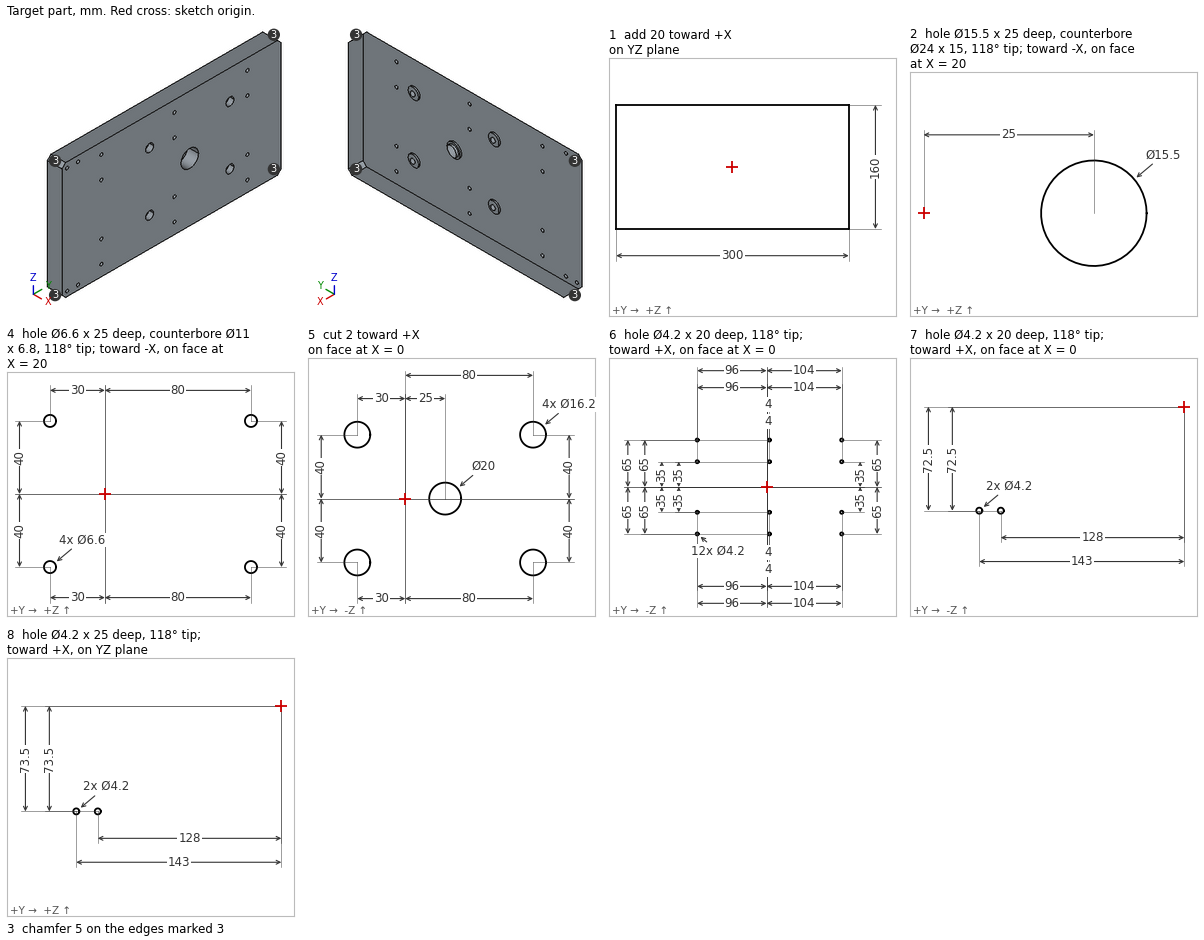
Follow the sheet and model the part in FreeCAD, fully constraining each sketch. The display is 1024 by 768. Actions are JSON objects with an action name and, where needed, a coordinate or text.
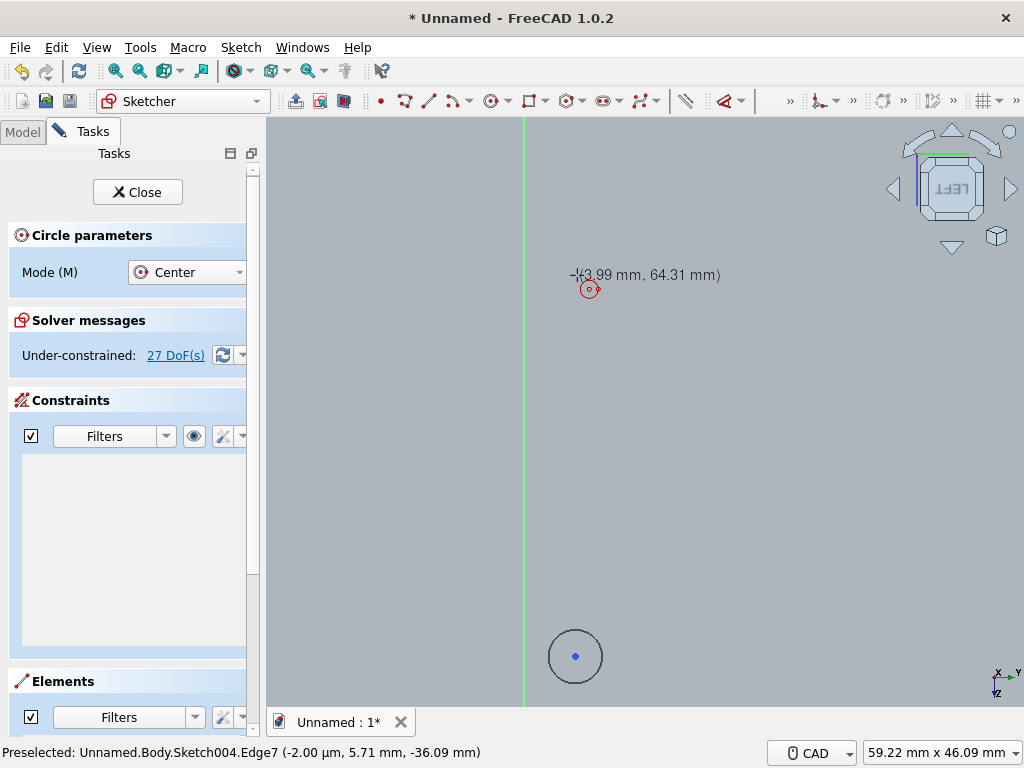
{"action": "scroll", "coordinate": [577, 275], "scroll_direction": "down", "scroll_amount": 9}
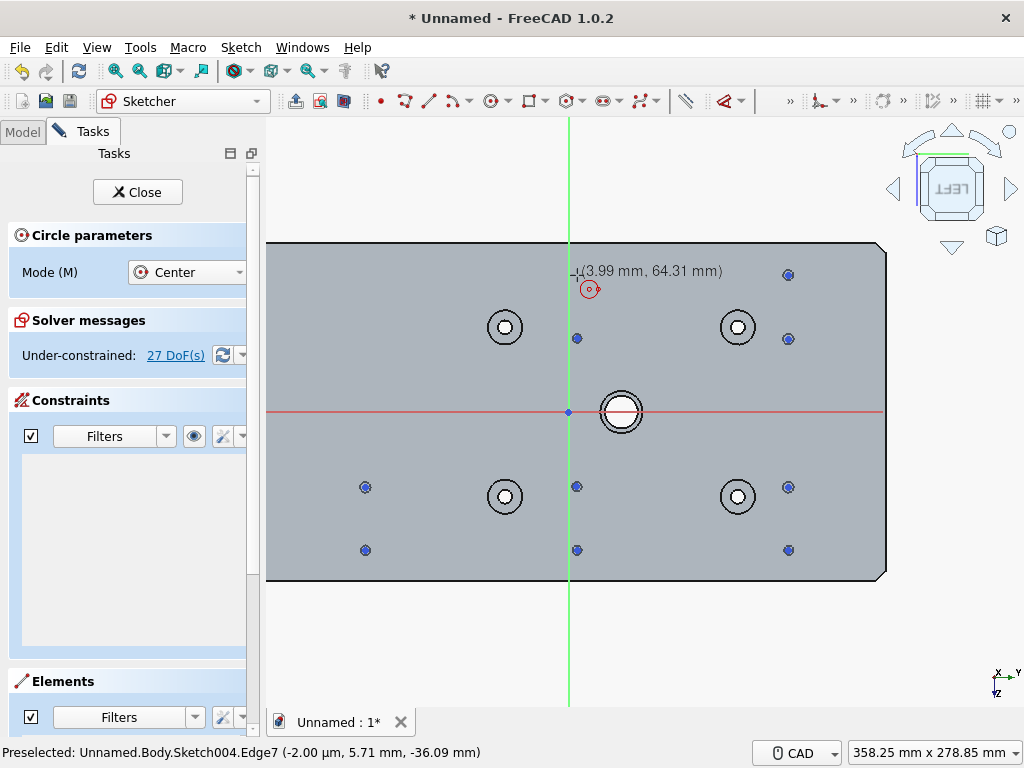
{"action": "scroll", "coordinate": [577, 275], "scroll_direction": "up", "scroll_amount": 4}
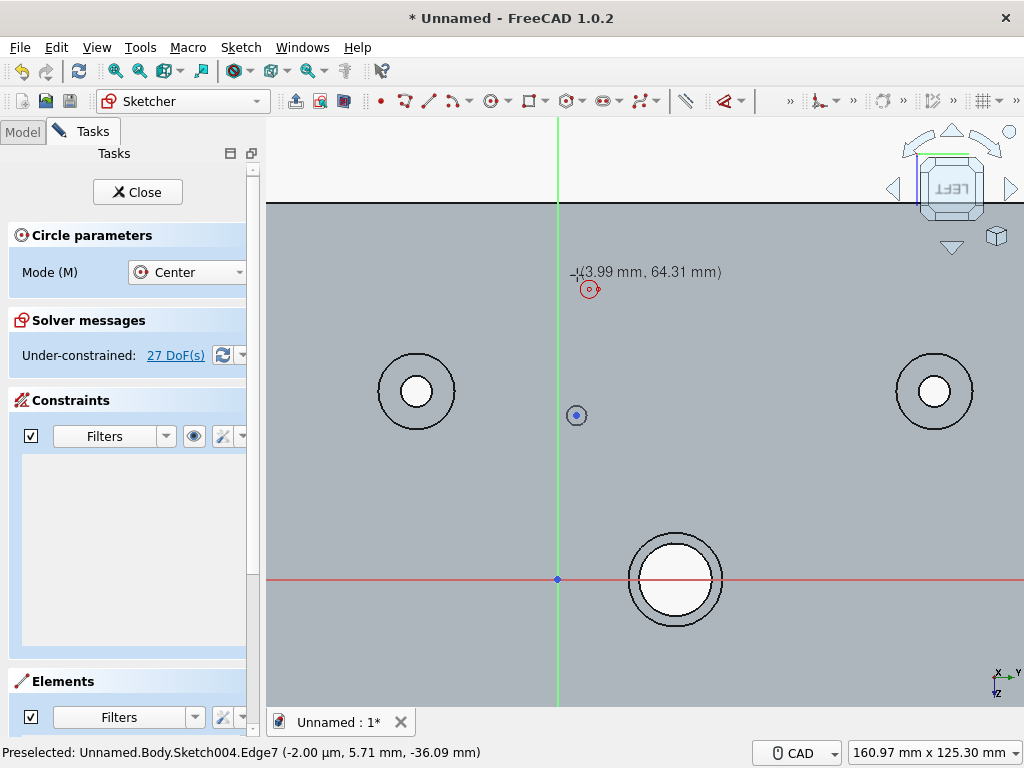
{"action": "left_click", "coordinate": [577, 274]}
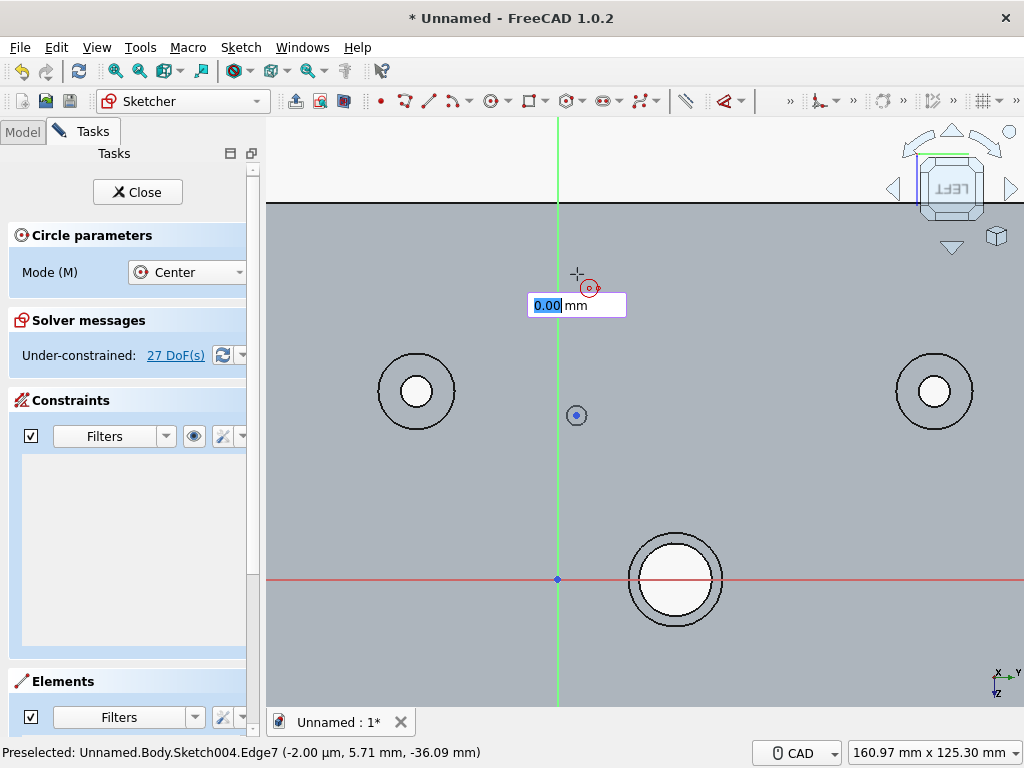
{"action": "scroll", "coordinate": [584, 267], "scroll_direction": "up", "scroll_amount": 3}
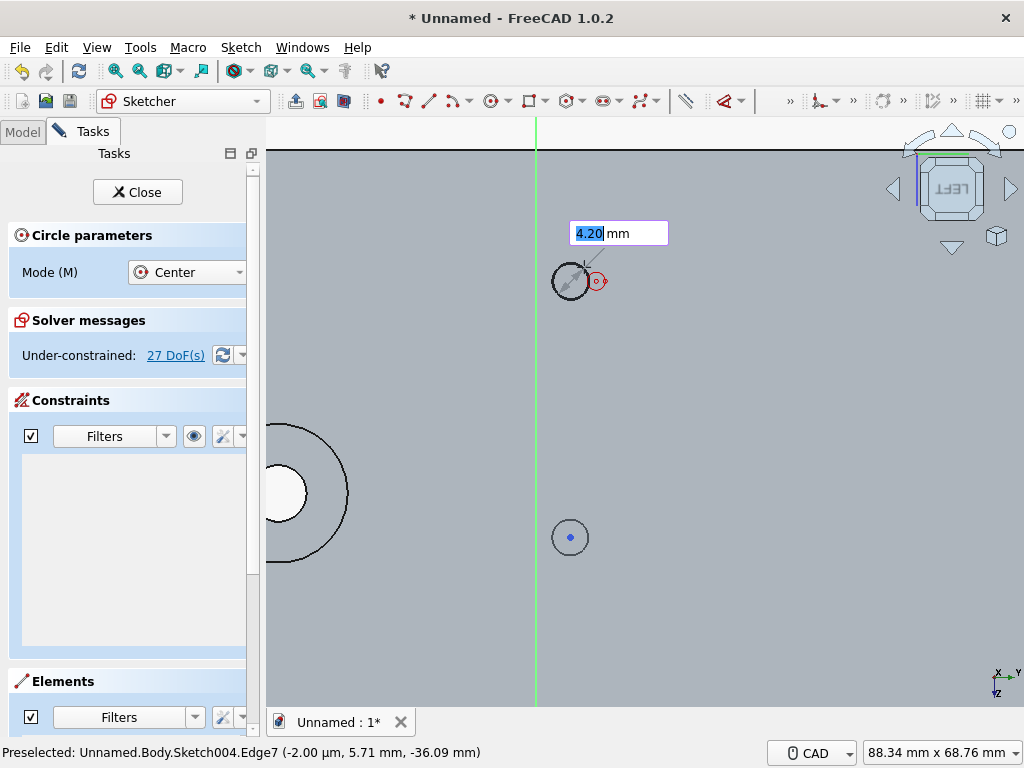
{"action": "left_click", "coordinate": [583, 266]}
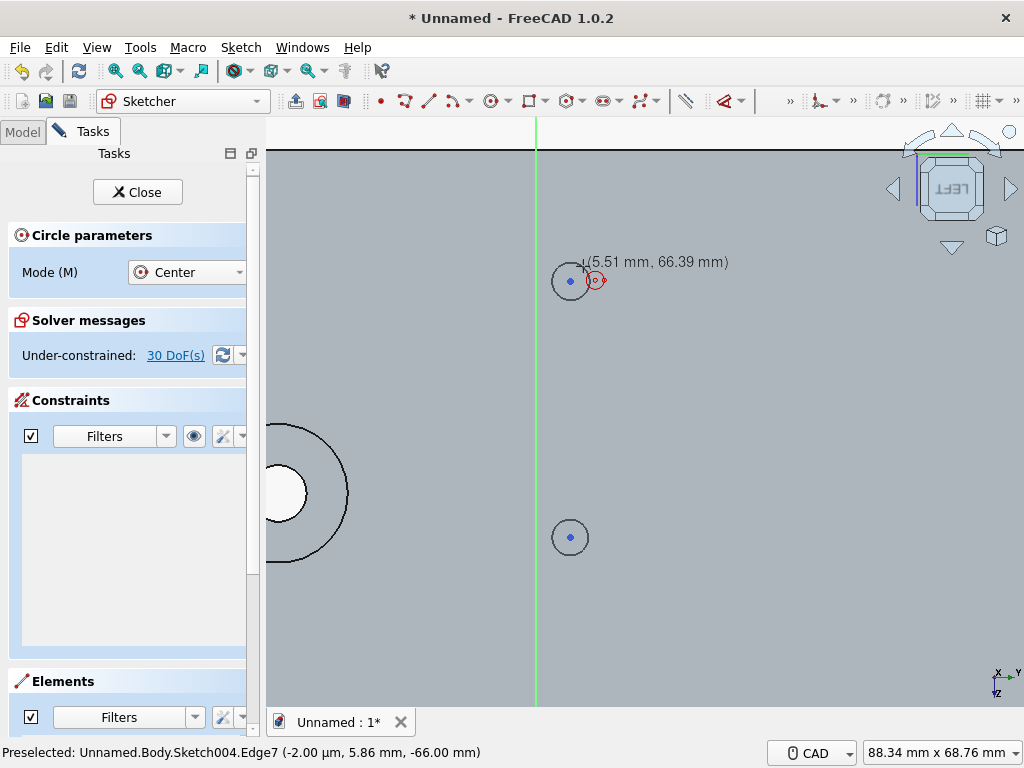
{"action": "scroll", "coordinate": [579, 273], "scroll_direction": "down", "scroll_amount": 7}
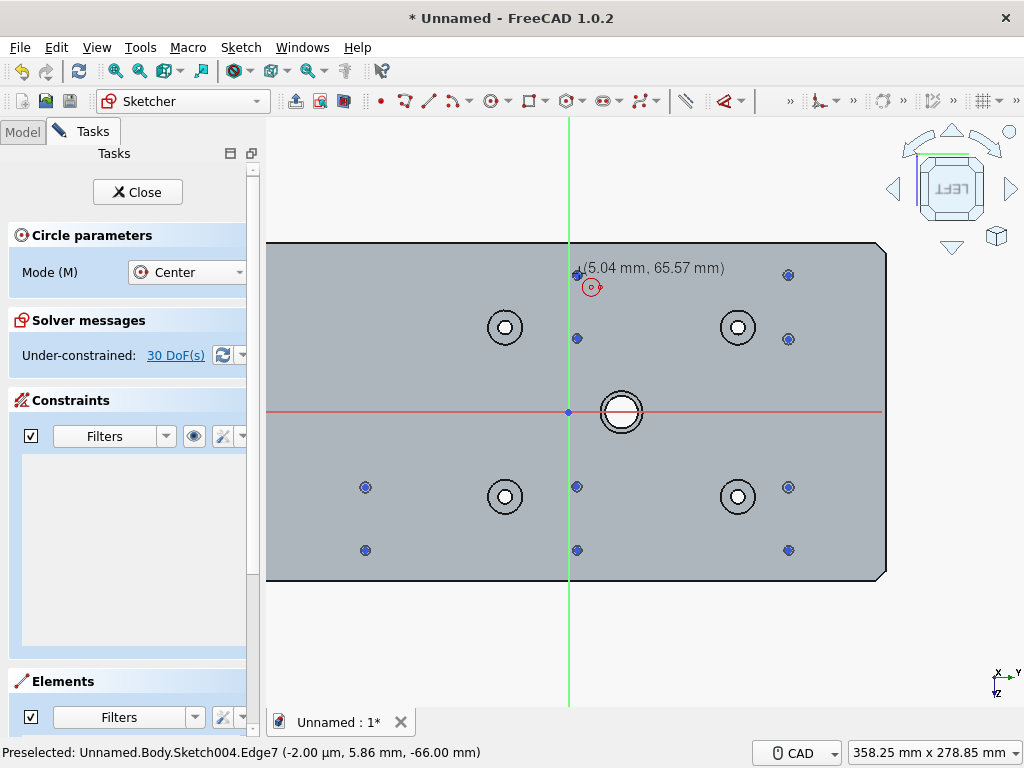
{"action": "scroll", "coordinate": [366, 338], "scroll_direction": "up", "scroll_amount": 9}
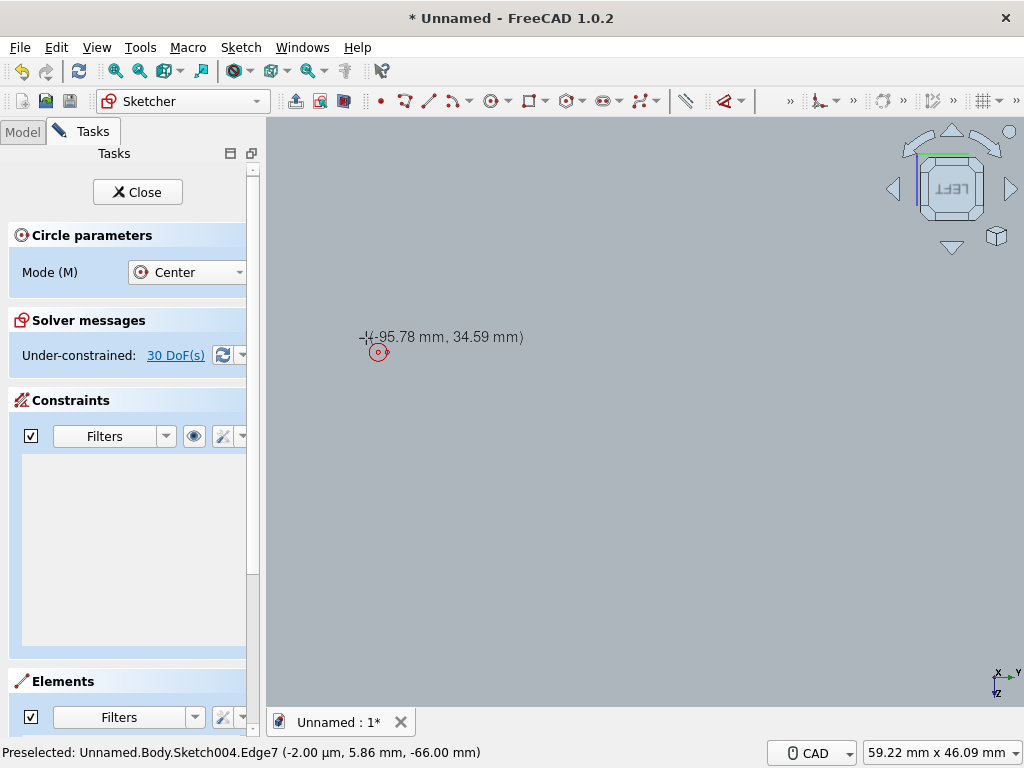
{"action": "scroll", "coordinate": [365, 338], "scroll_direction": "down", "scroll_amount": 9}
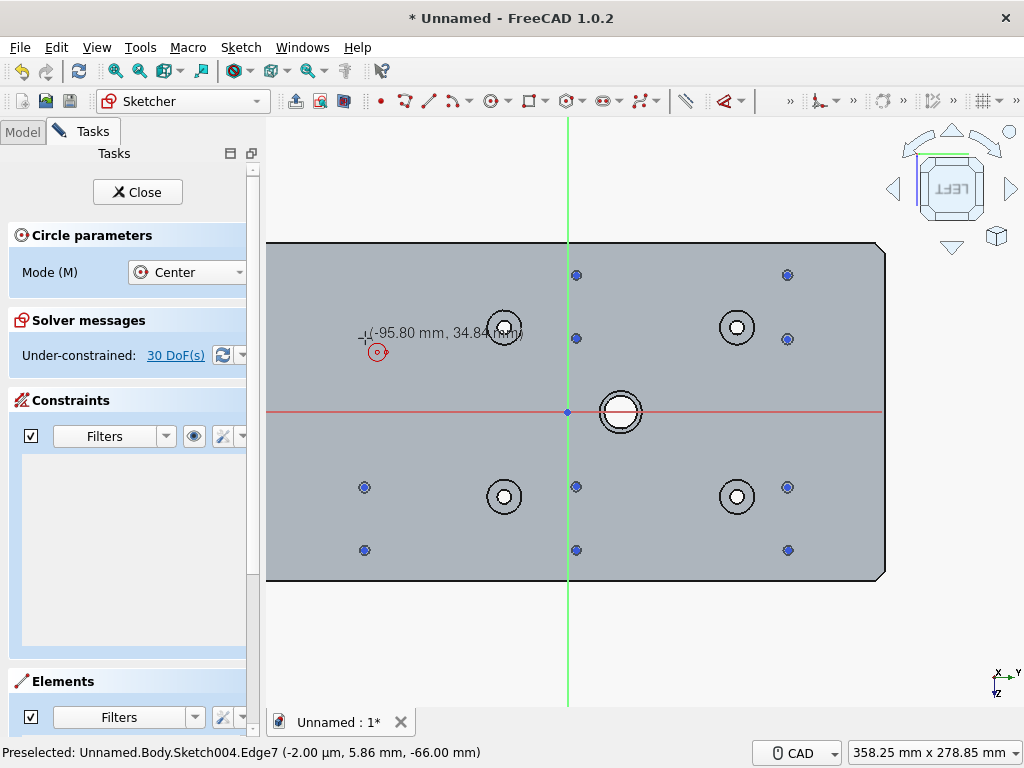
{"action": "left_click", "coordinate": [365, 338]}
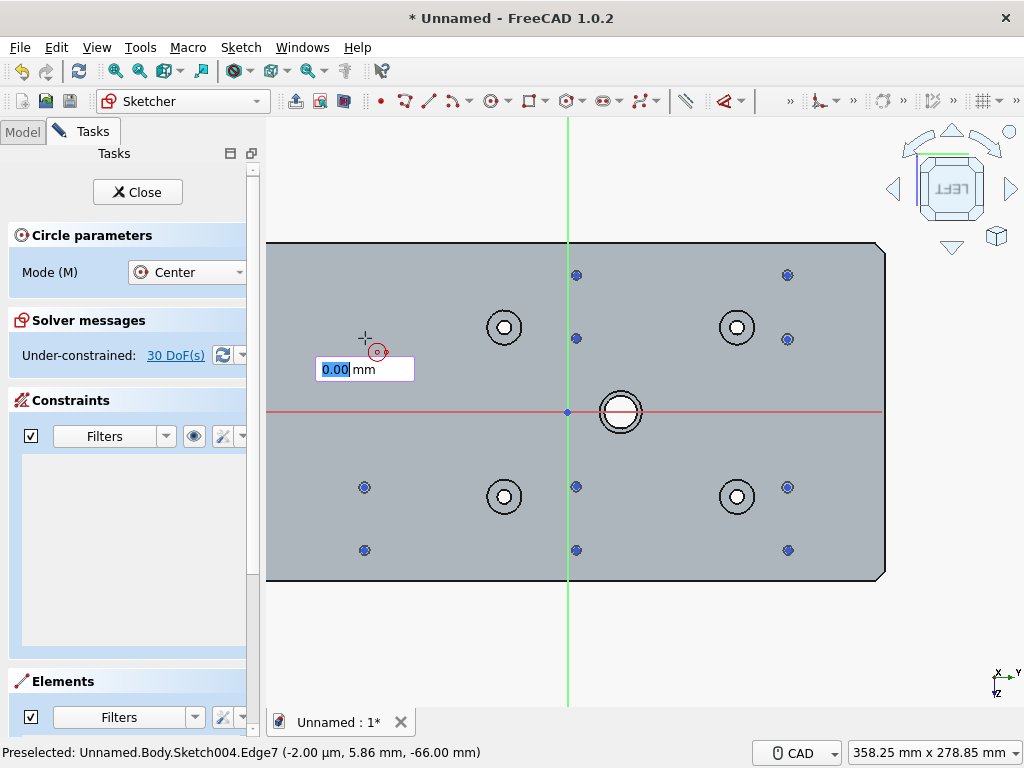
{"action": "scroll", "coordinate": [368, 335], "scroll_direction": "up", "scroll_amount": 7}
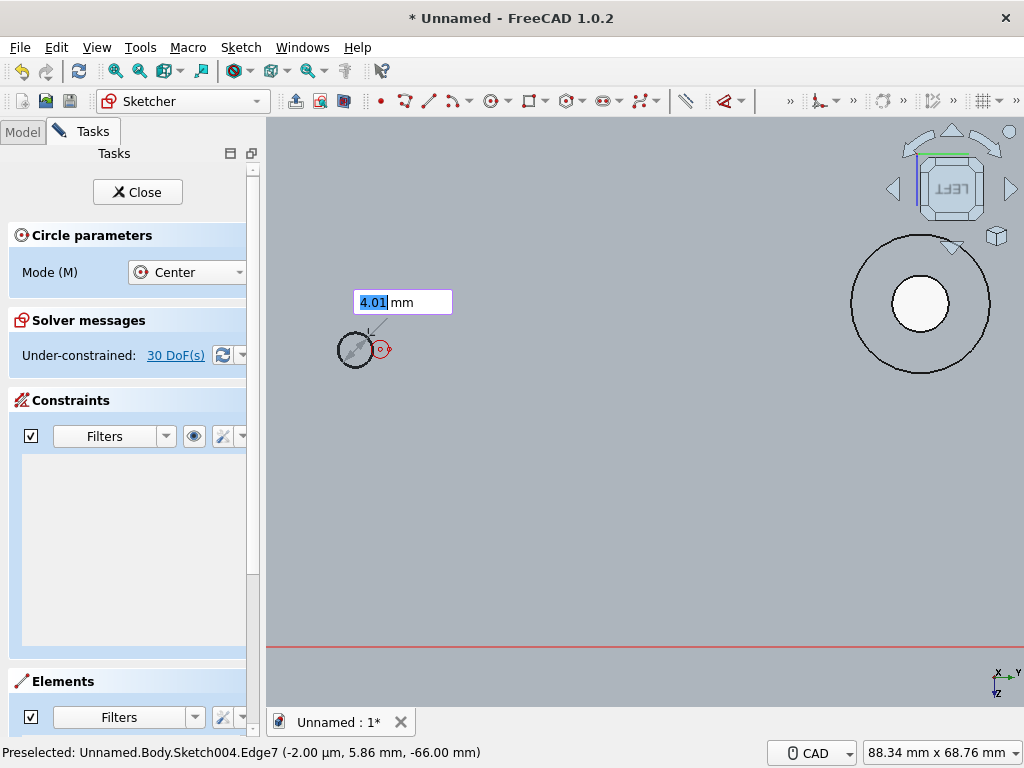
{"action": "left_click", "coordinate": [367, 334]}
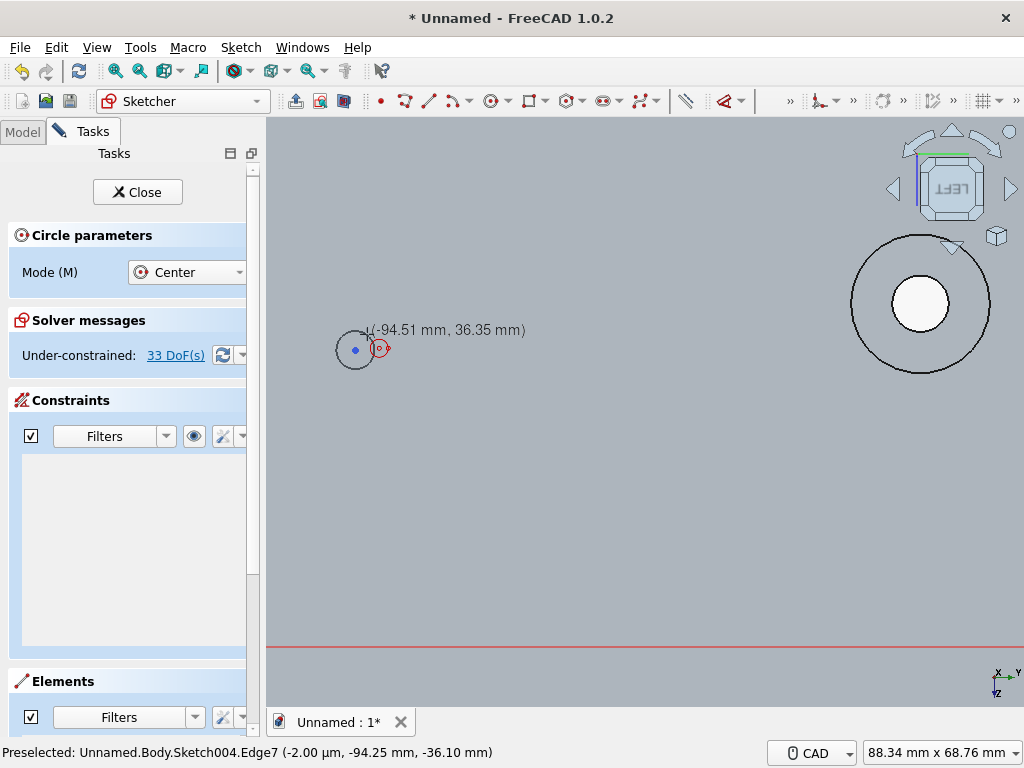
{"action": "scroll", "coordinate": [368, 335], "scroll_direction": "down", "scroll_amount": 7}